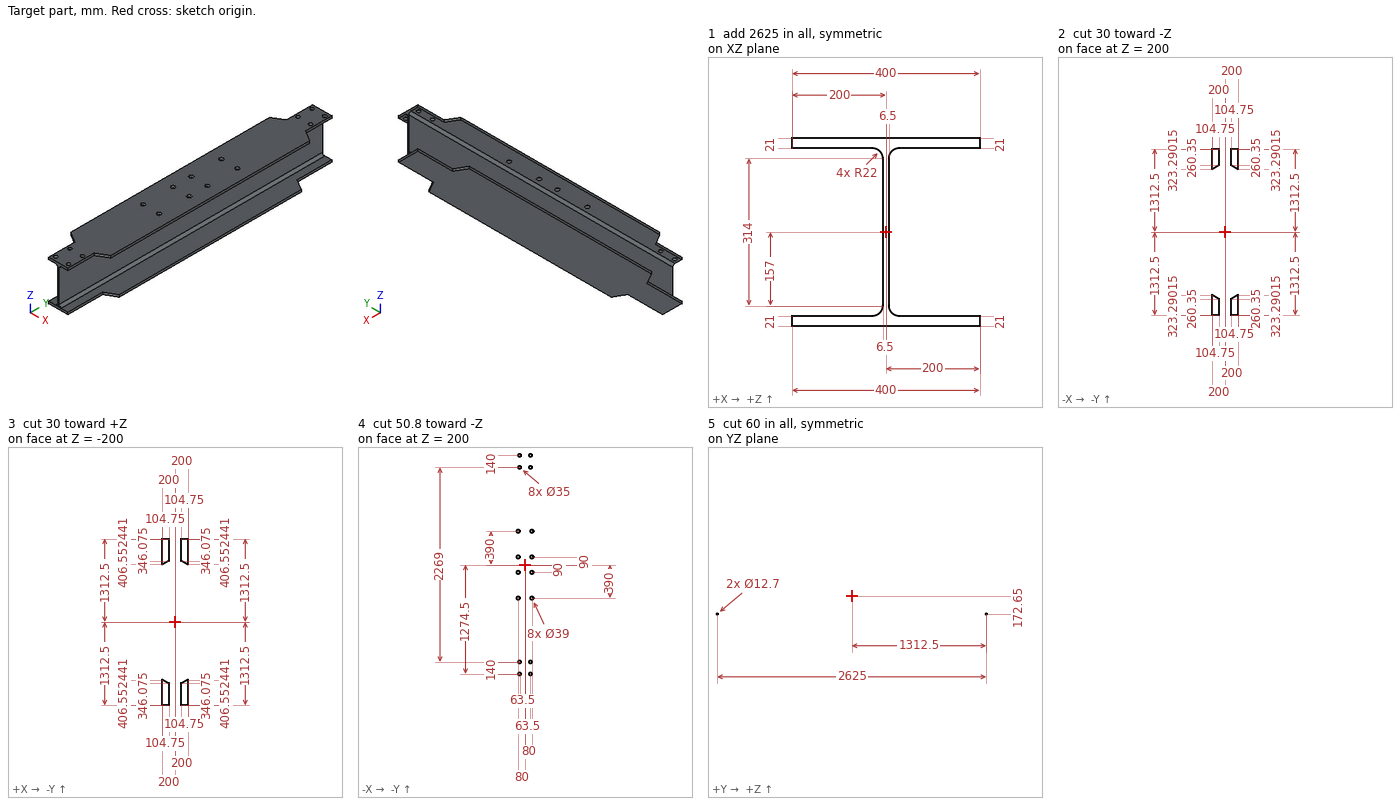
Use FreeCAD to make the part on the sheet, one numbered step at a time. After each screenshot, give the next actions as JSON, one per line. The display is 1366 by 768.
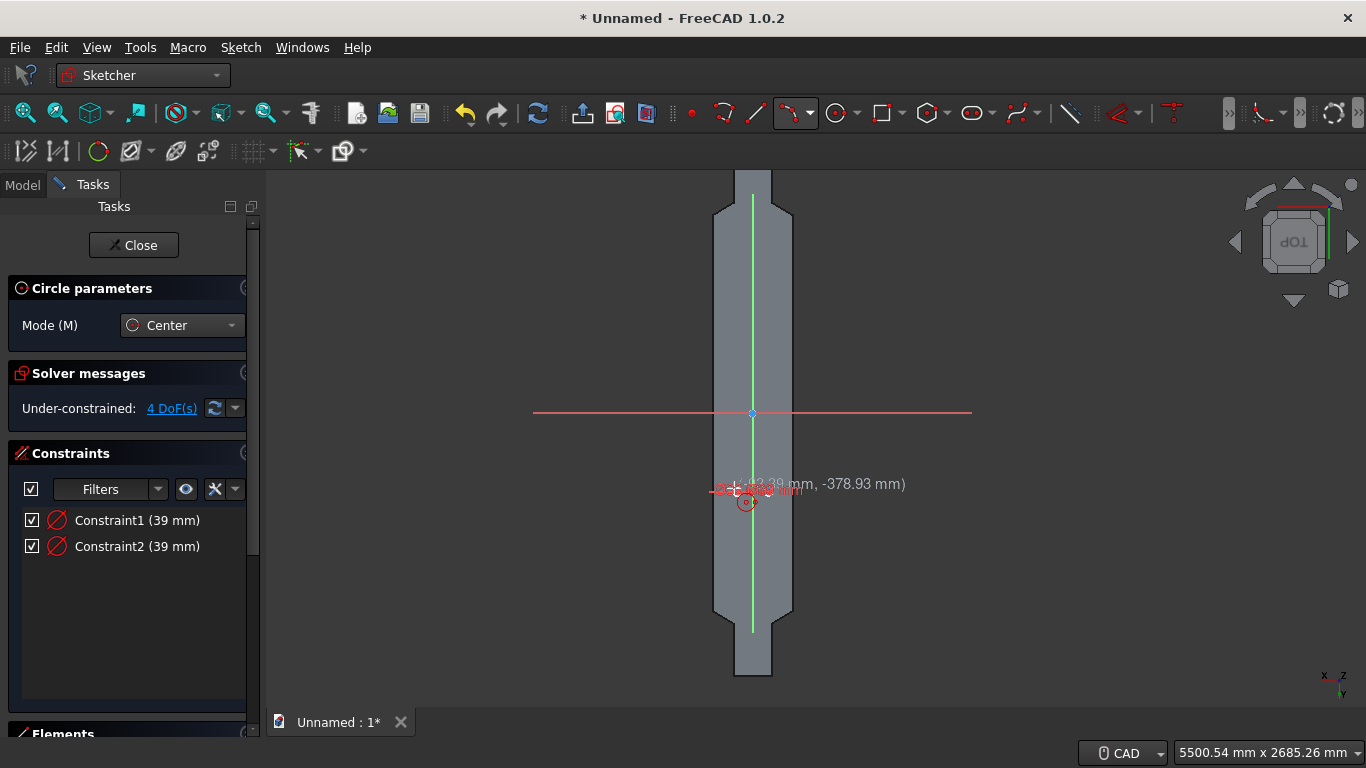
{"action": "scroll", "coordinate": [737, 335], "scroll_direction": "up", "scroll_amount": 9}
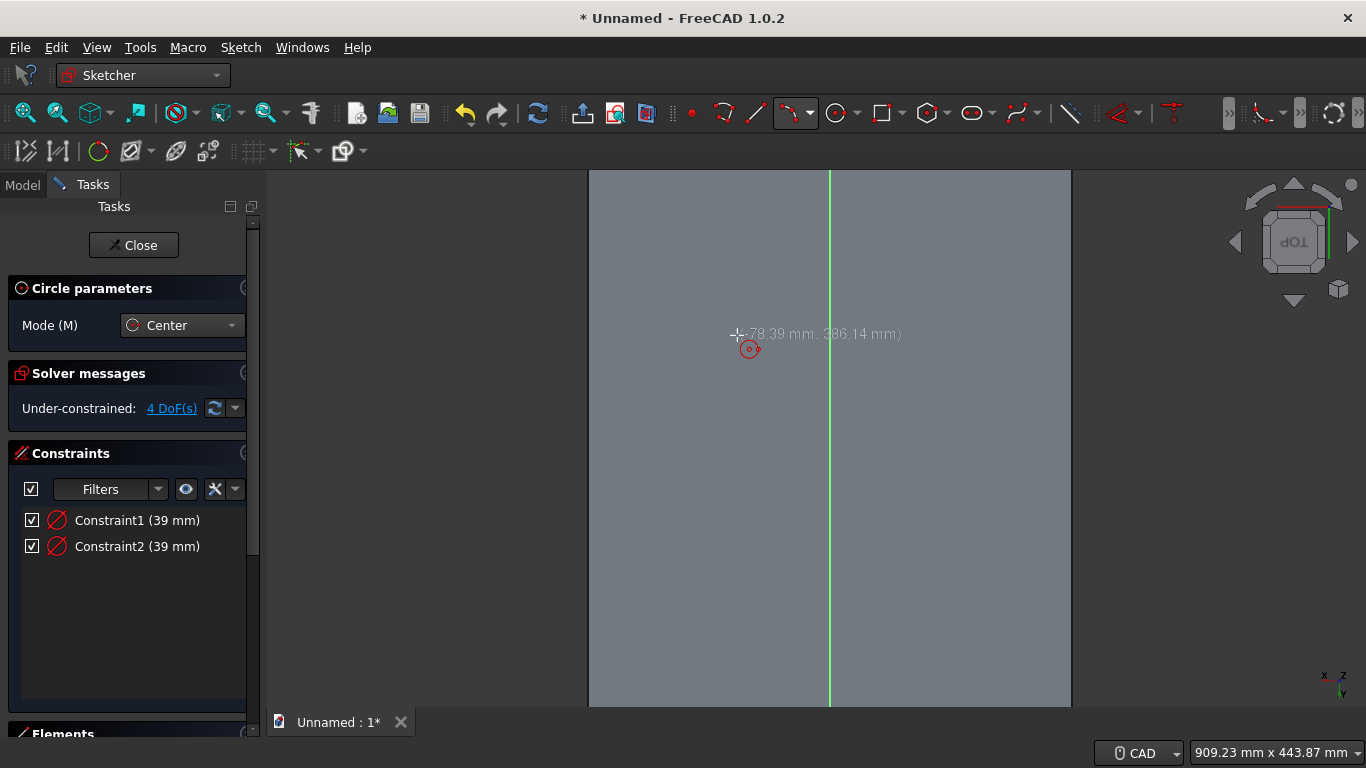
{"action": "scroll", "coordinate": [737, 393], "scroll_direction": "down", "scroll_amount": 11}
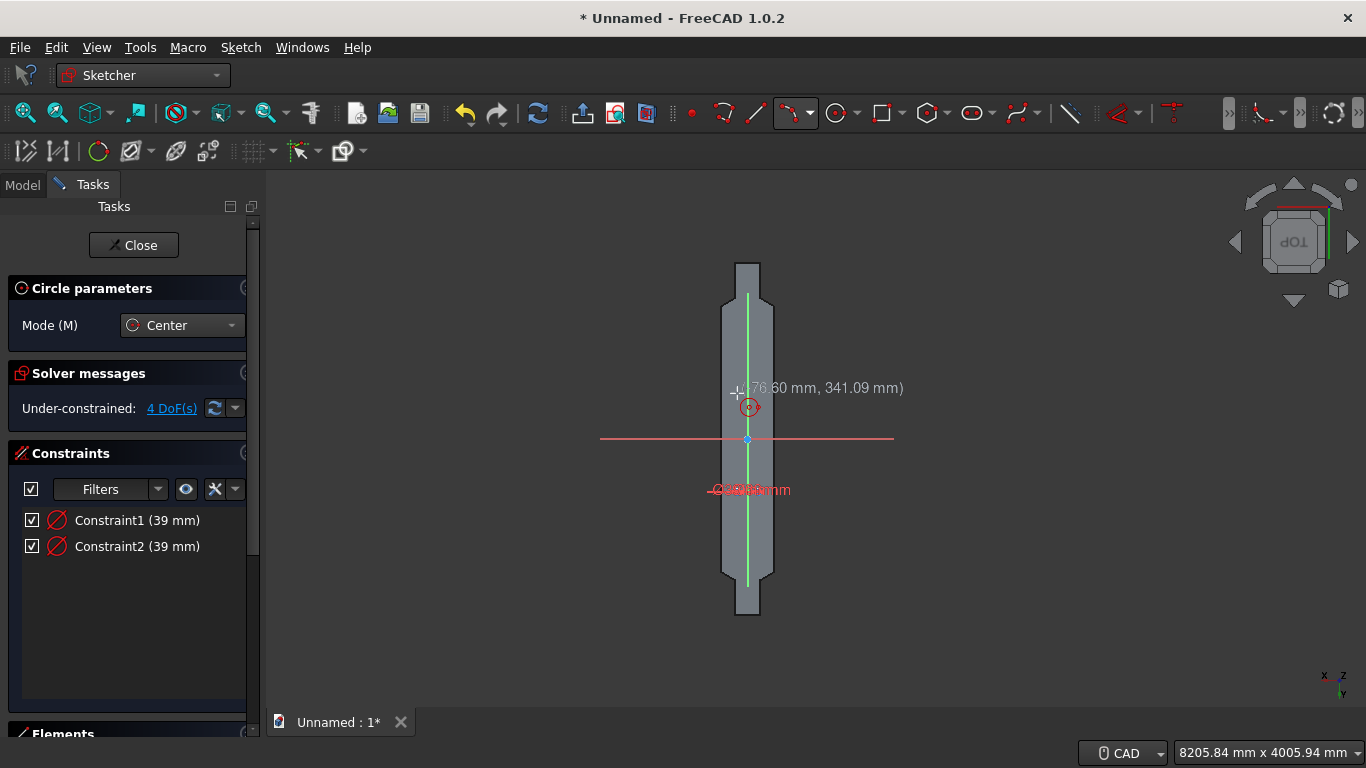
{"action": "scroll", "coordinate": [737, 387], "scroll_direction": "up", "scroll_amount": 2}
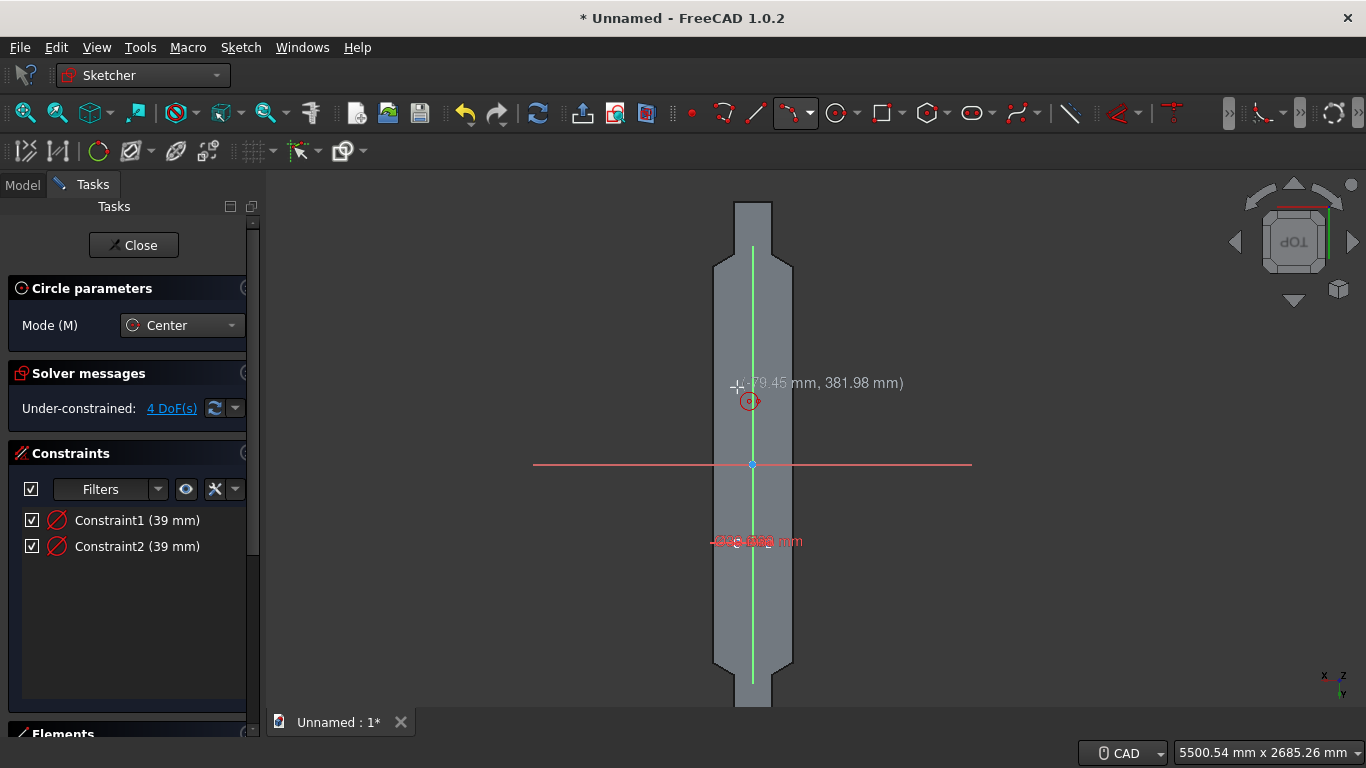
{"action": "left_click", "coordinate": [737, 387]}
{"action": "mouse_move", "coordinate": [734, 384]}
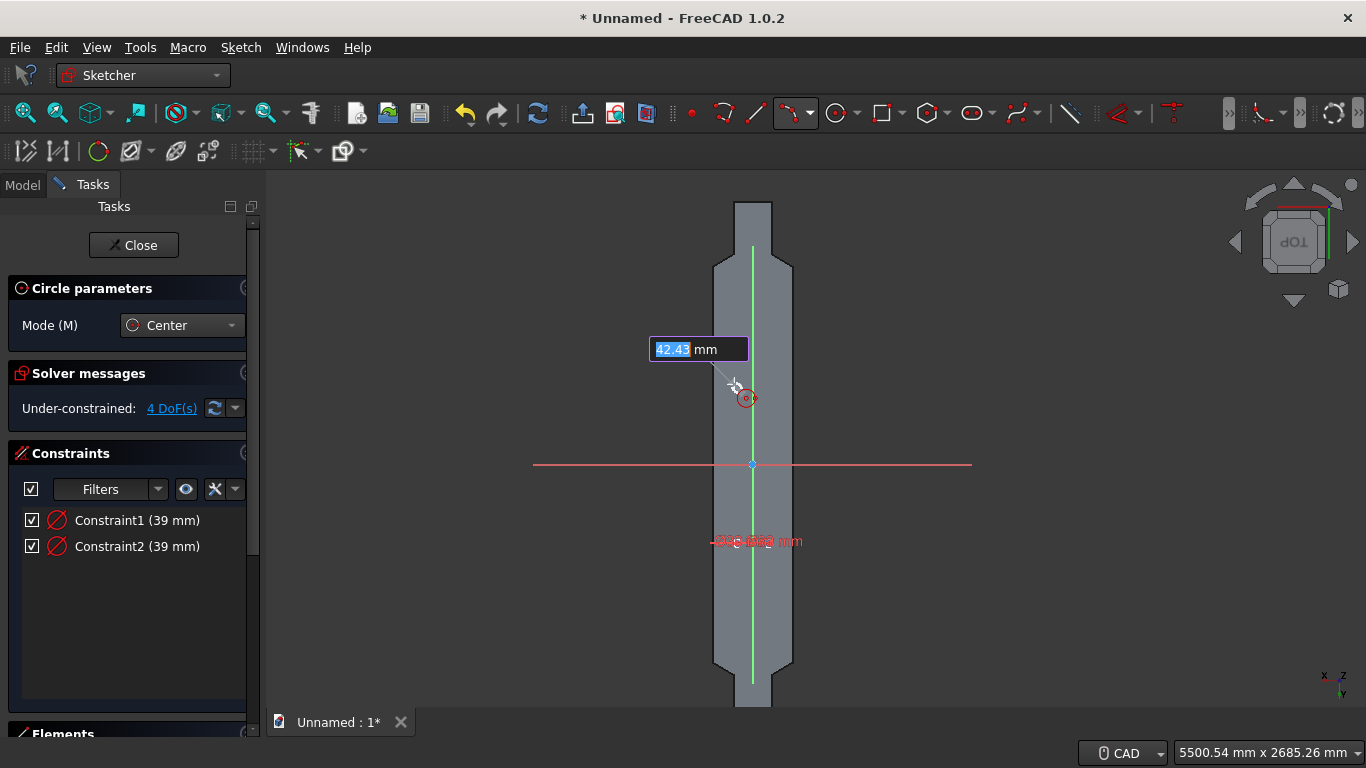
{"action": "type", "text": "39"}
{"action": "key", "text": "Return"}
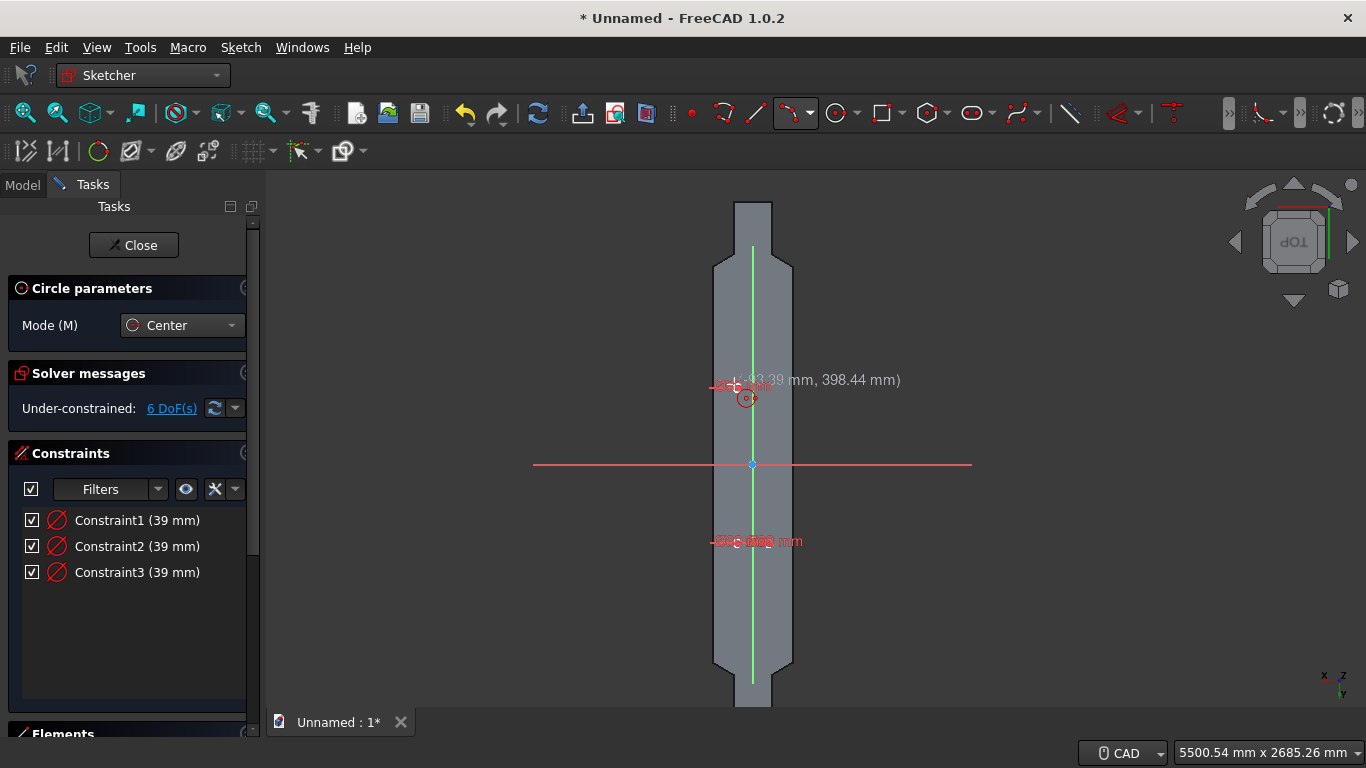
{"action": "scroll", "coordinate": [769, 387], "scroll_direction": "up", "scroll_amount": 9}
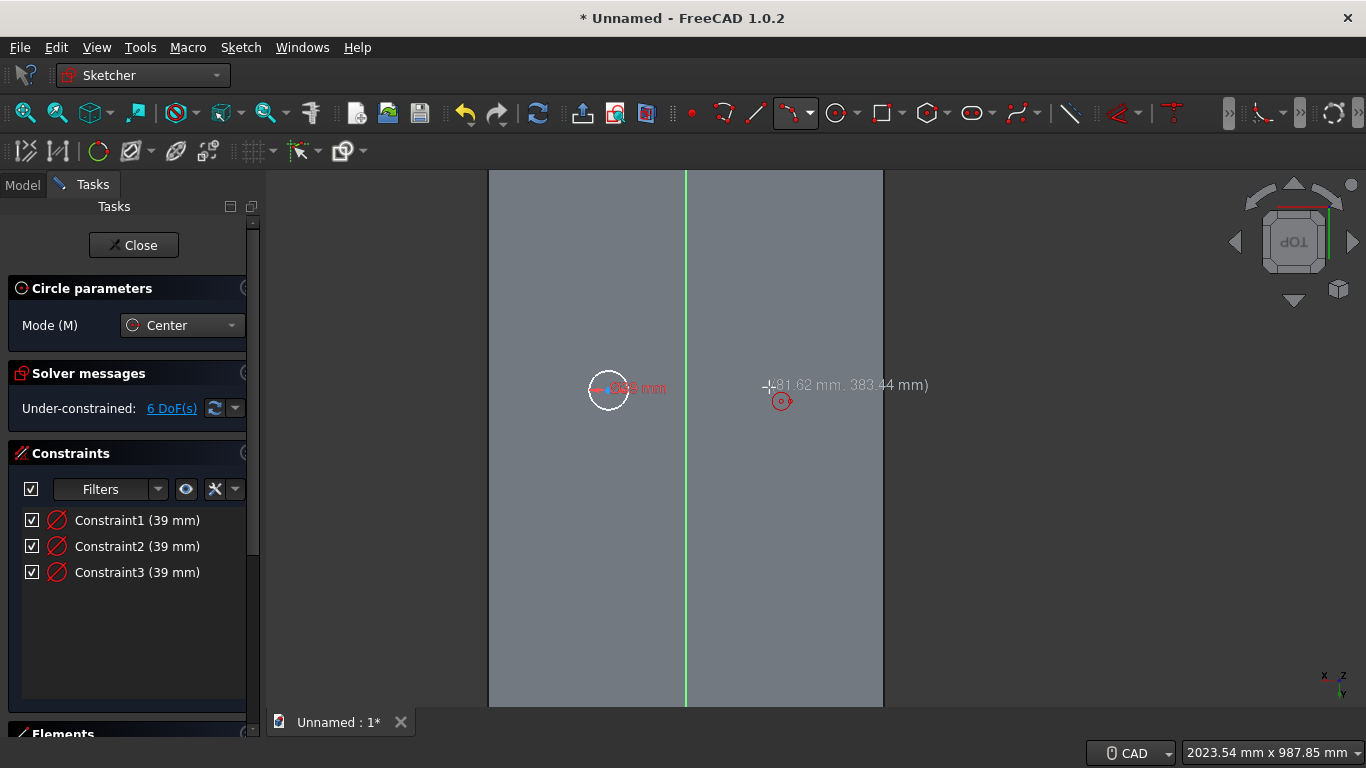
{"action": "scroll", "coordinate": [757, 387], "scroll_direction": "down", "scroll_amount": 11}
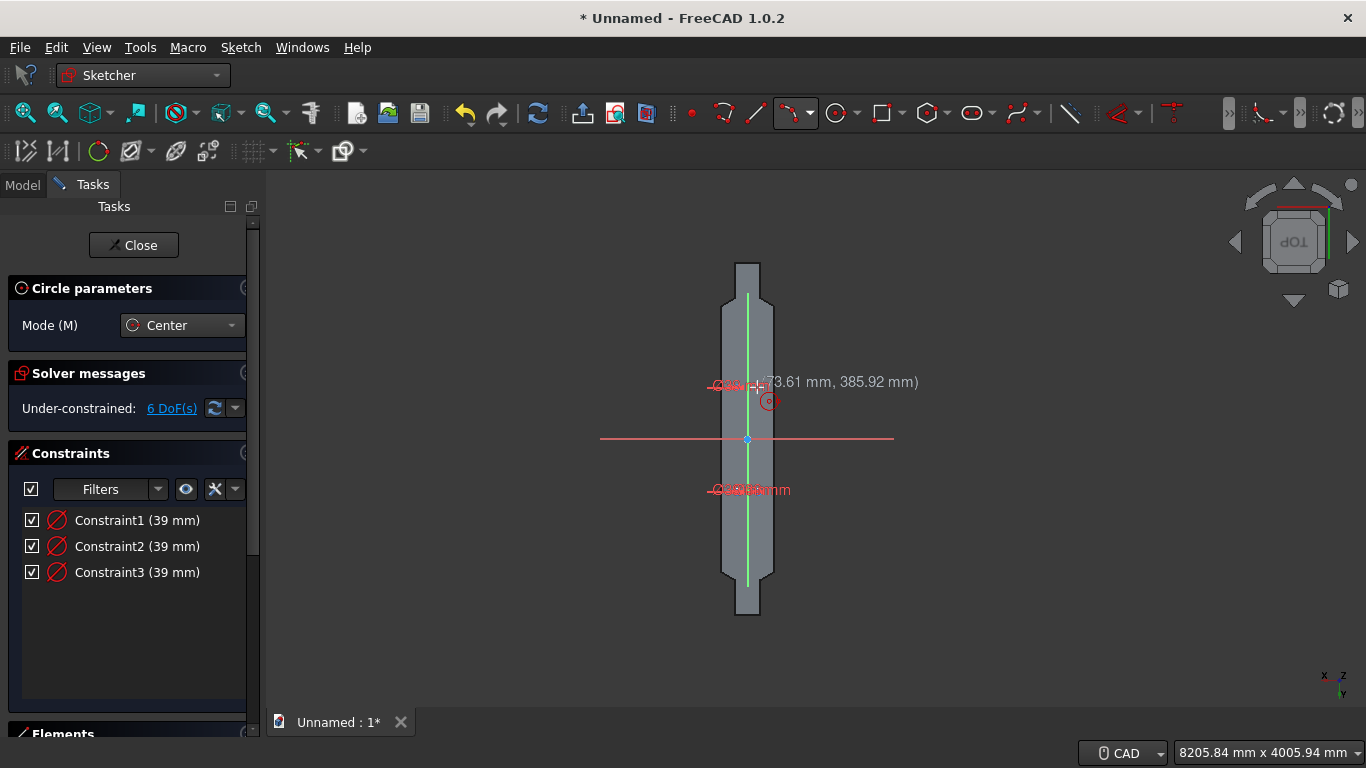
{"action": "scroll", "coordinate": [758, 387], "scroll_direction": "up", "scroll_amount": 2}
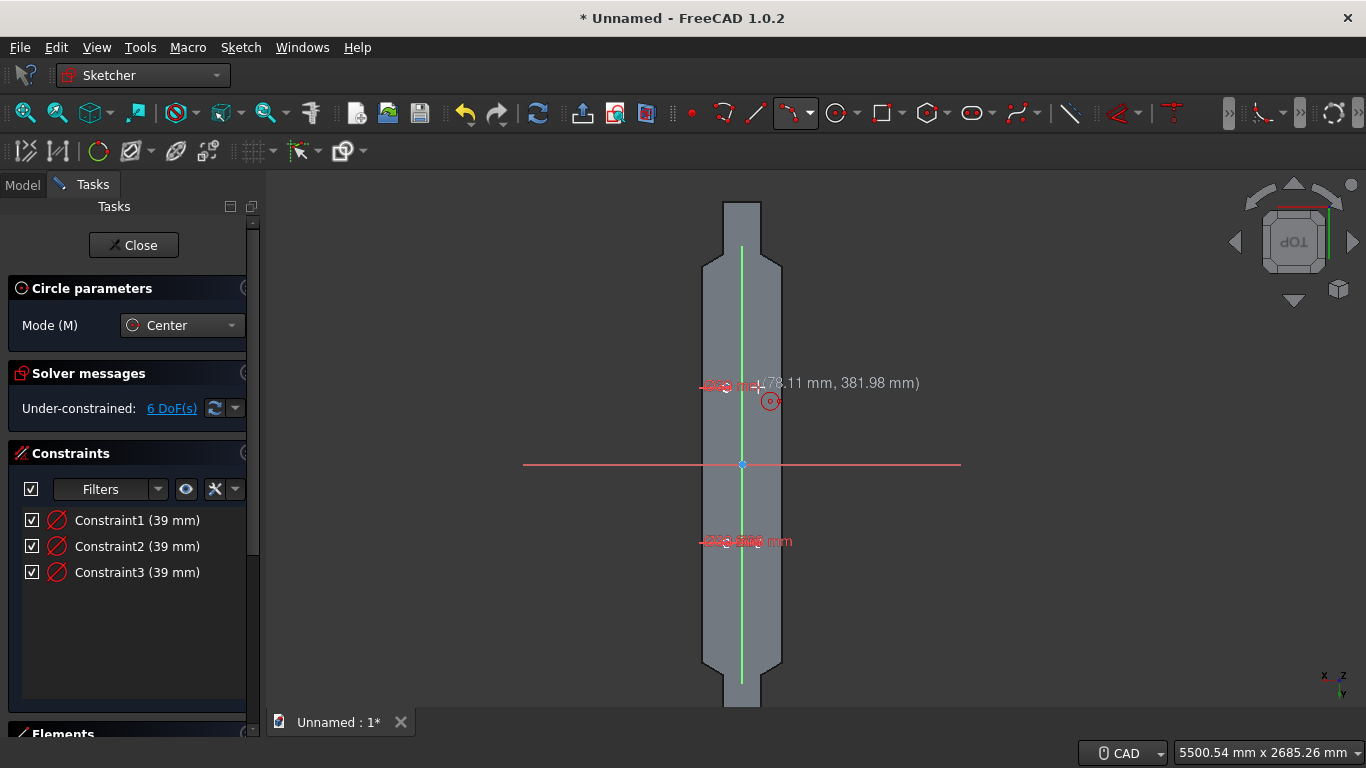
{"action": "left_click", "coordinate": [758, 387]}
{"action": "mouse_move", "coordinate": [761, 384]}